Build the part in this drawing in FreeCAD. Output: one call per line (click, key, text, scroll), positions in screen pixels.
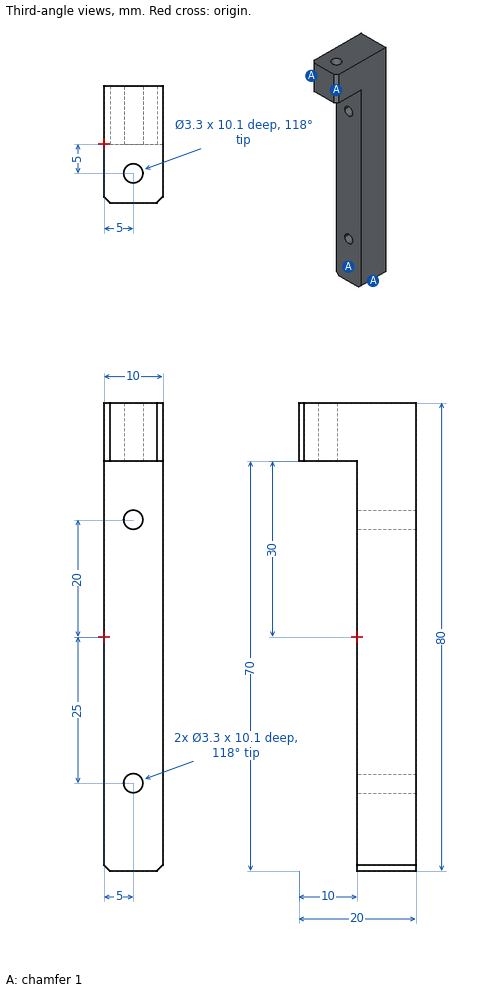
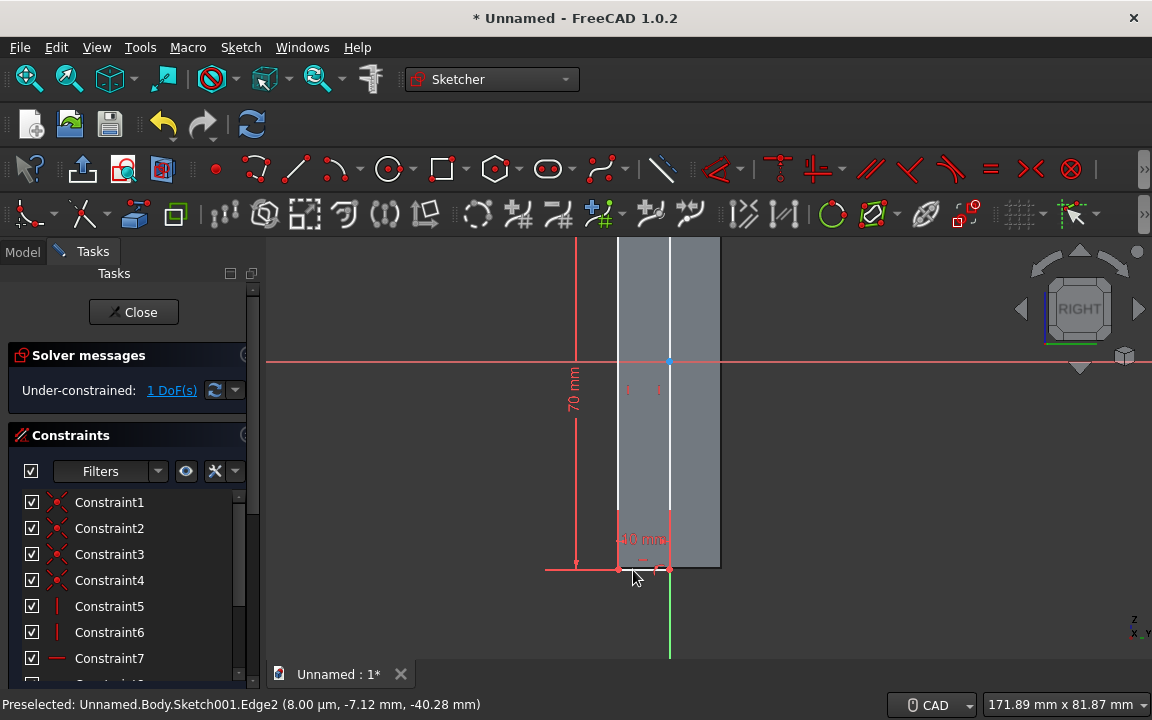
scroll(634, 570, down, 2)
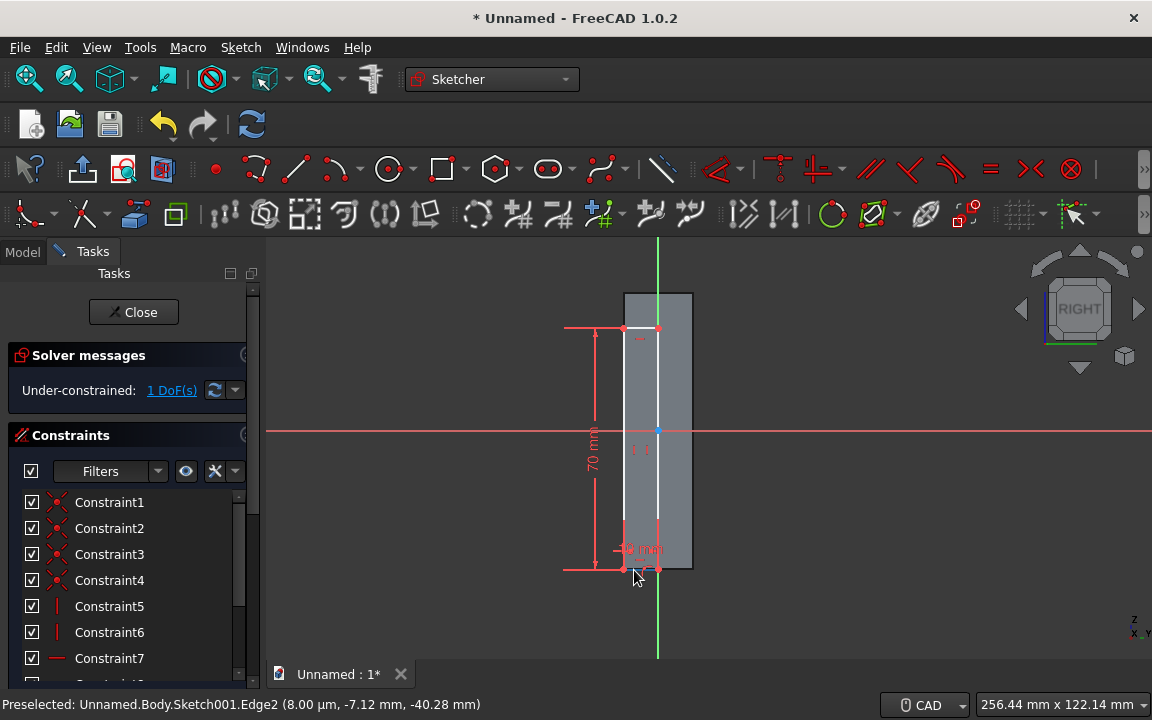
click(624, 328)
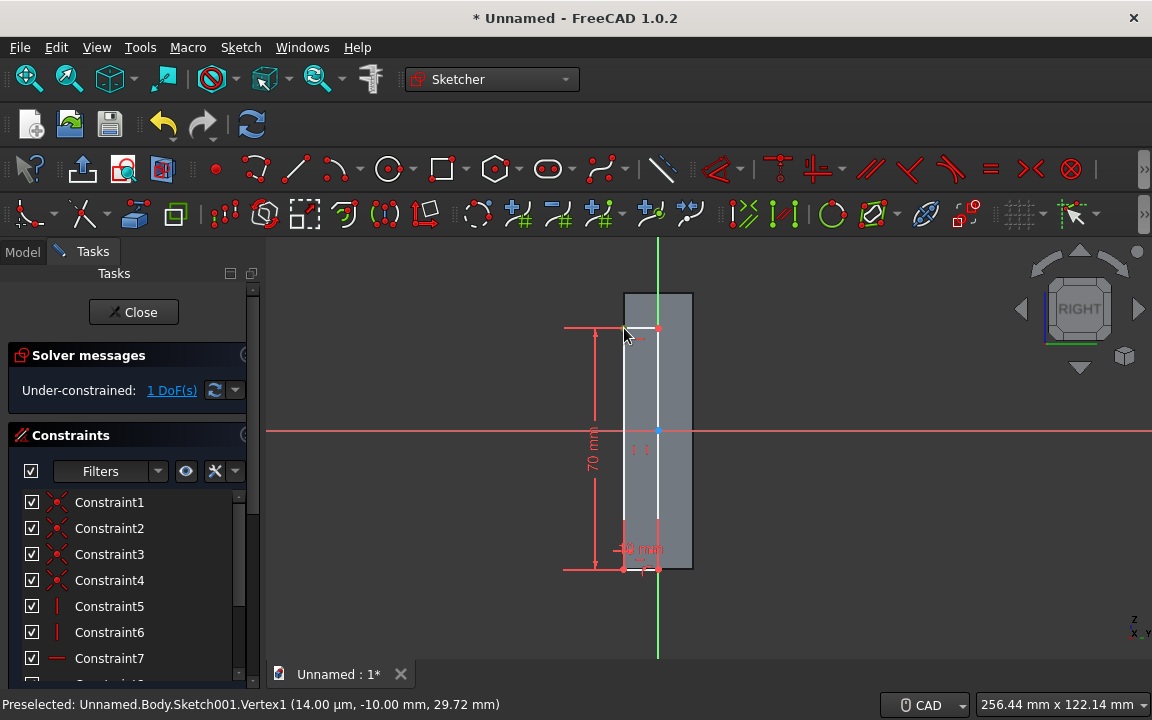
key(i)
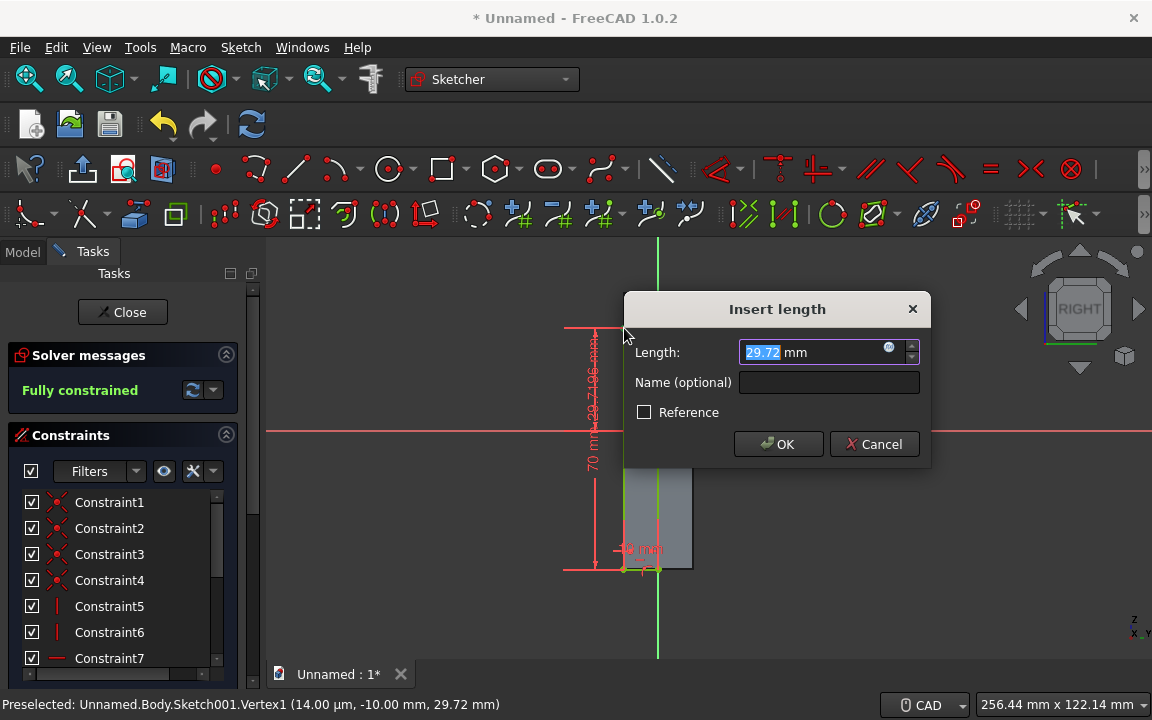
text(30)
key(Return)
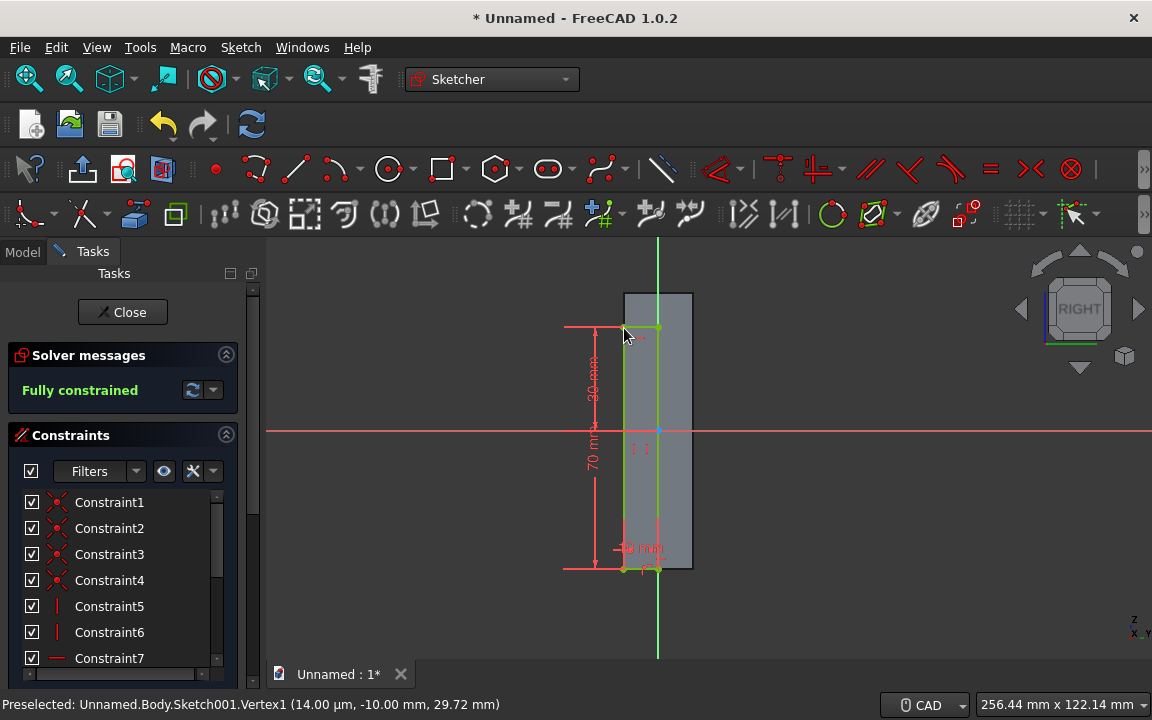
click(123, 312)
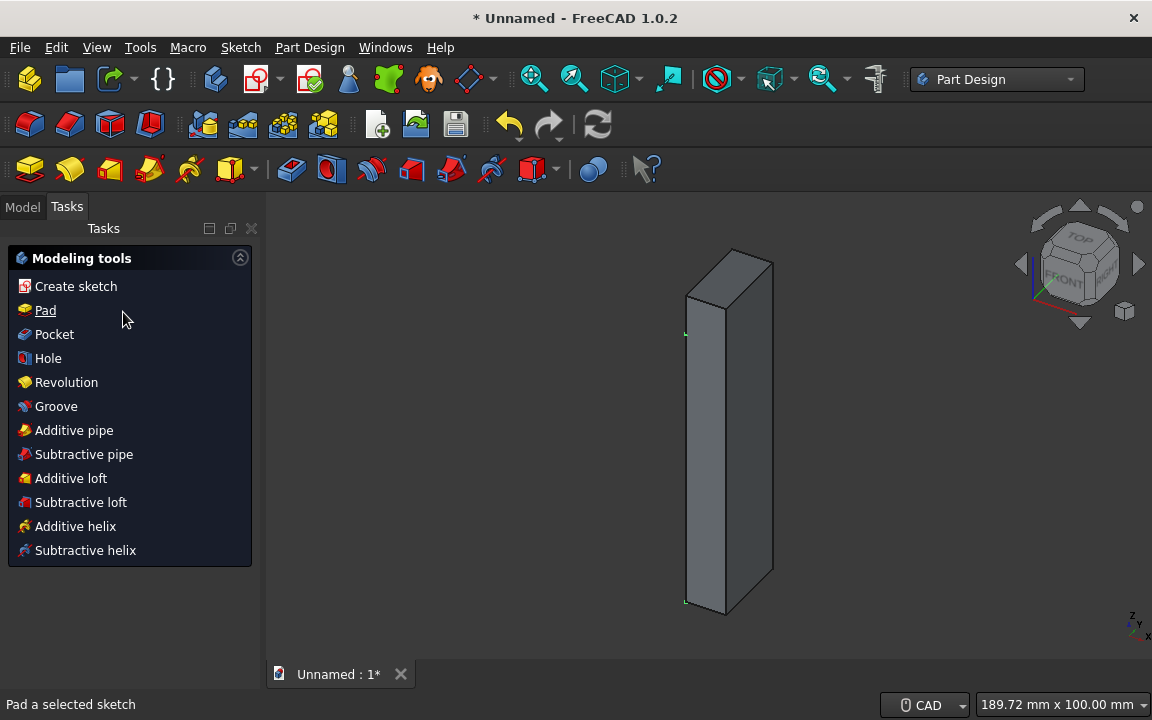
click(292, 170)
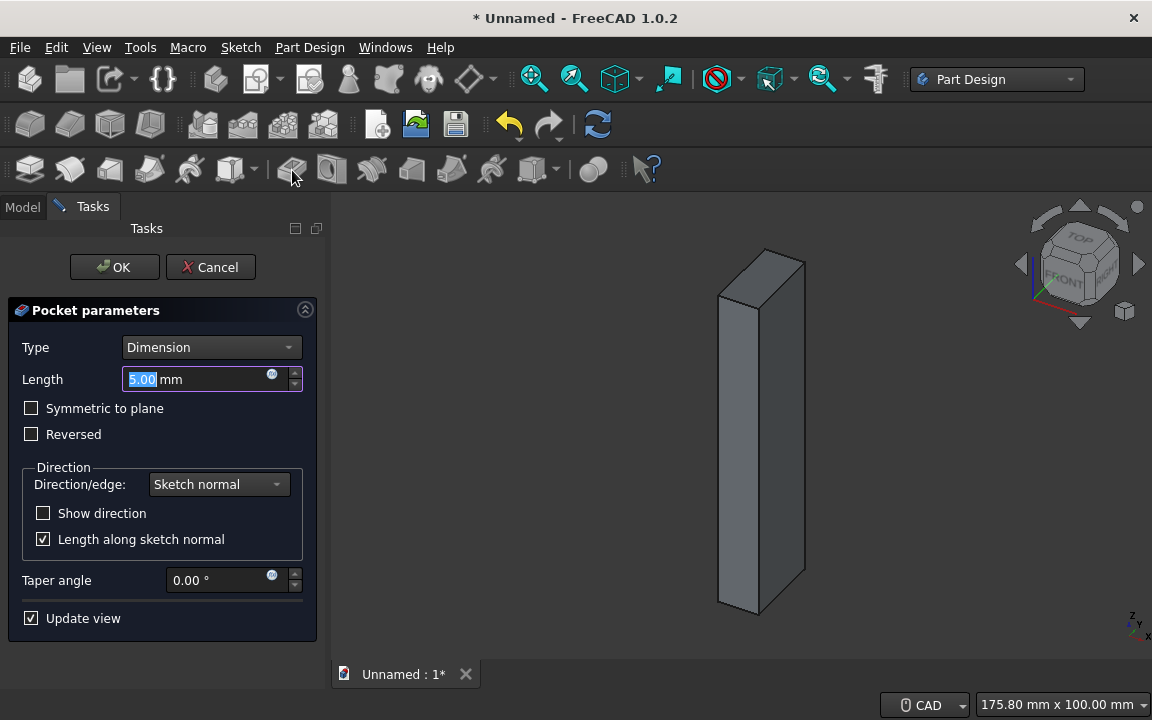
click(212, 348)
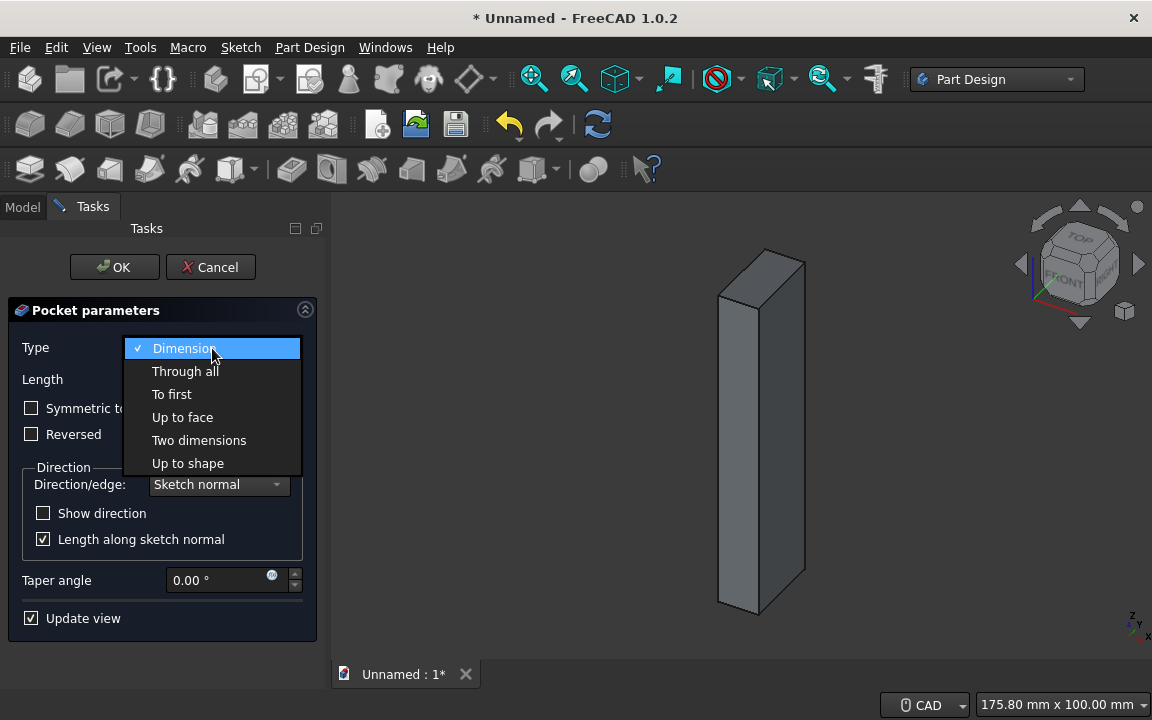
click(212, 372)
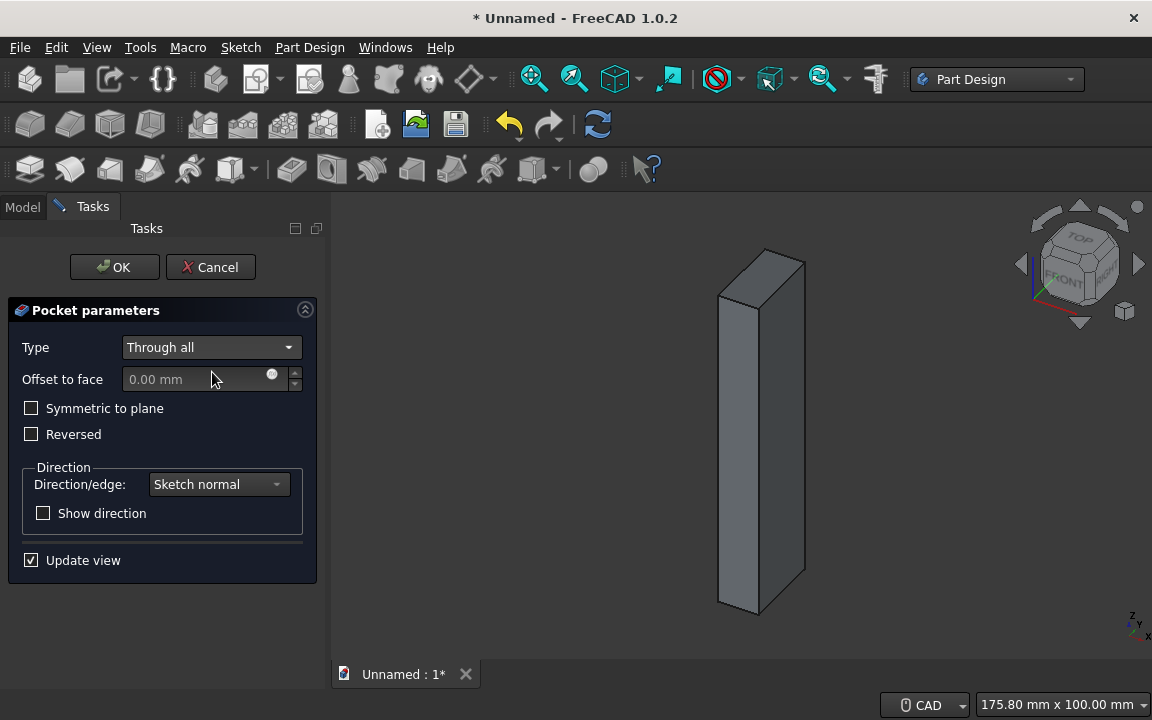
click(30, 434)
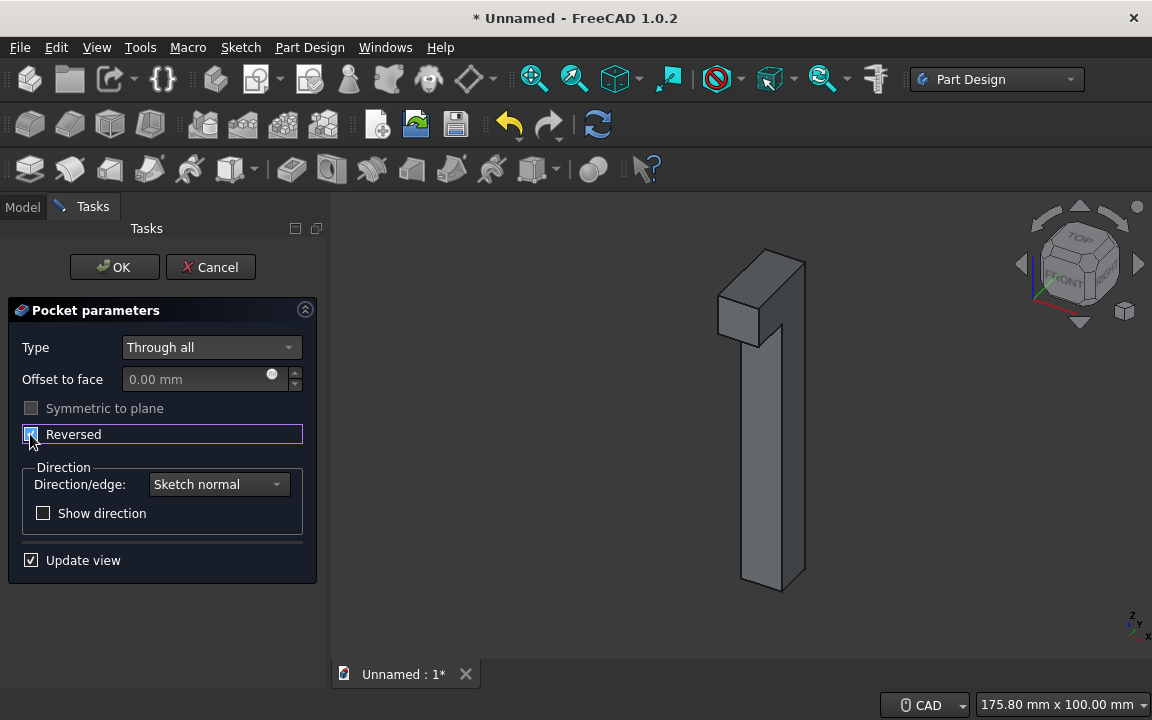
click(115, 267)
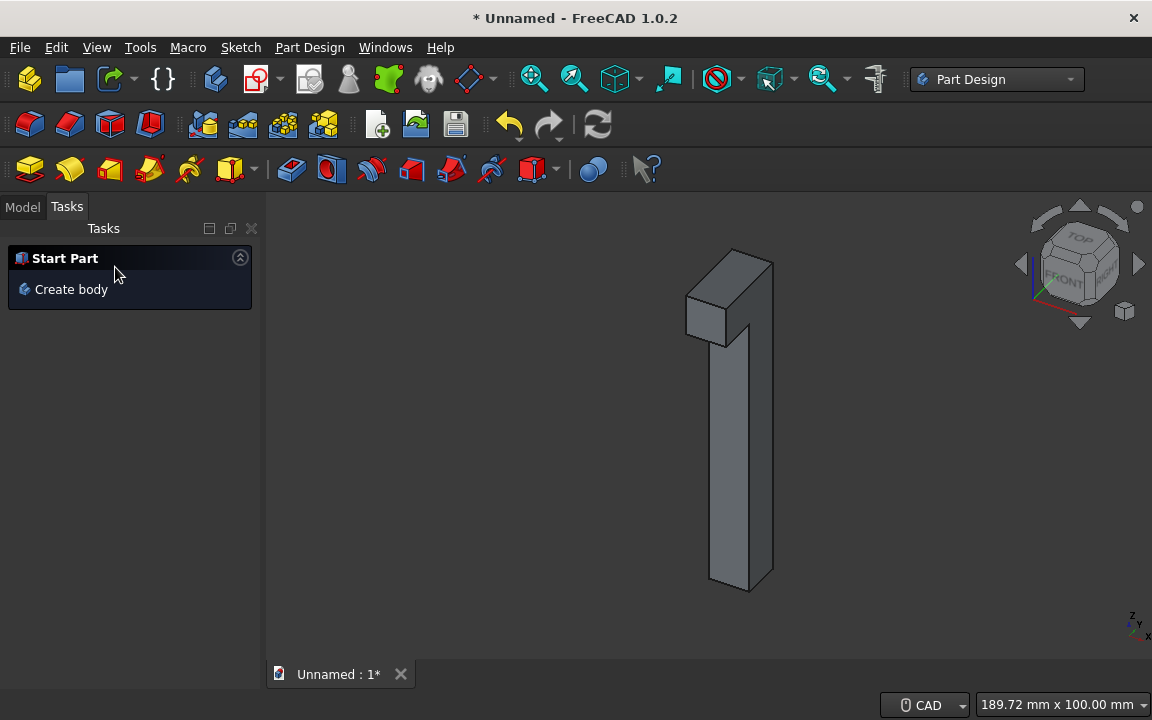
key(5)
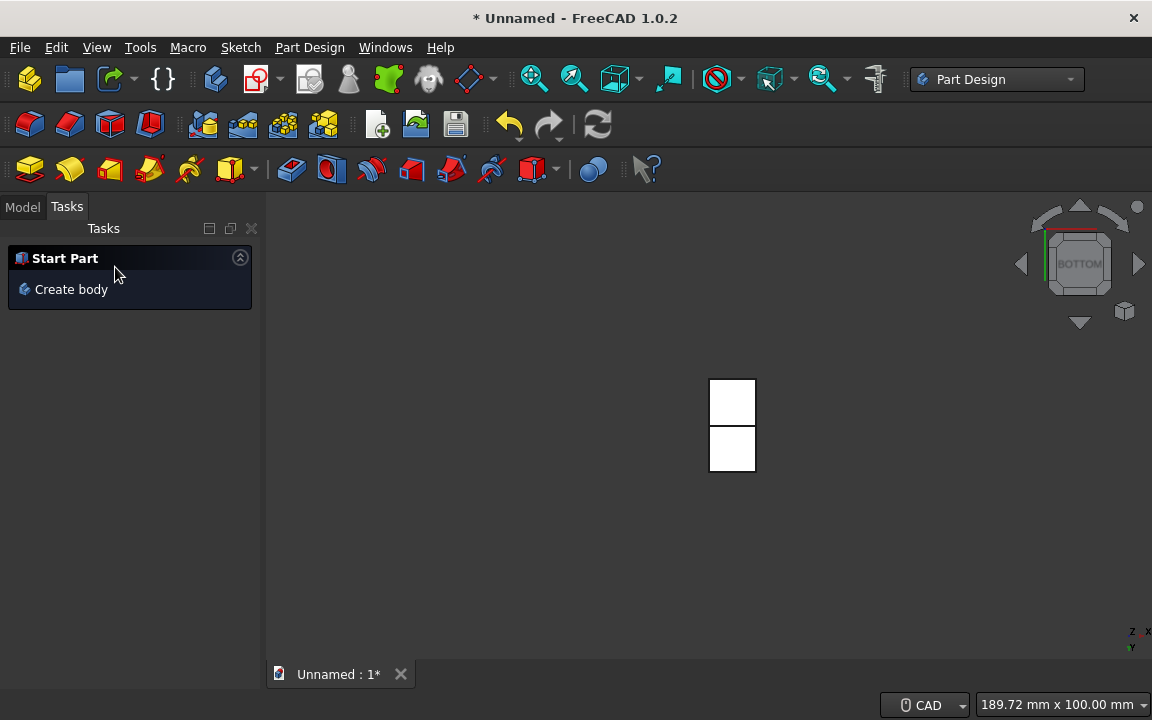
key(v)
key(f)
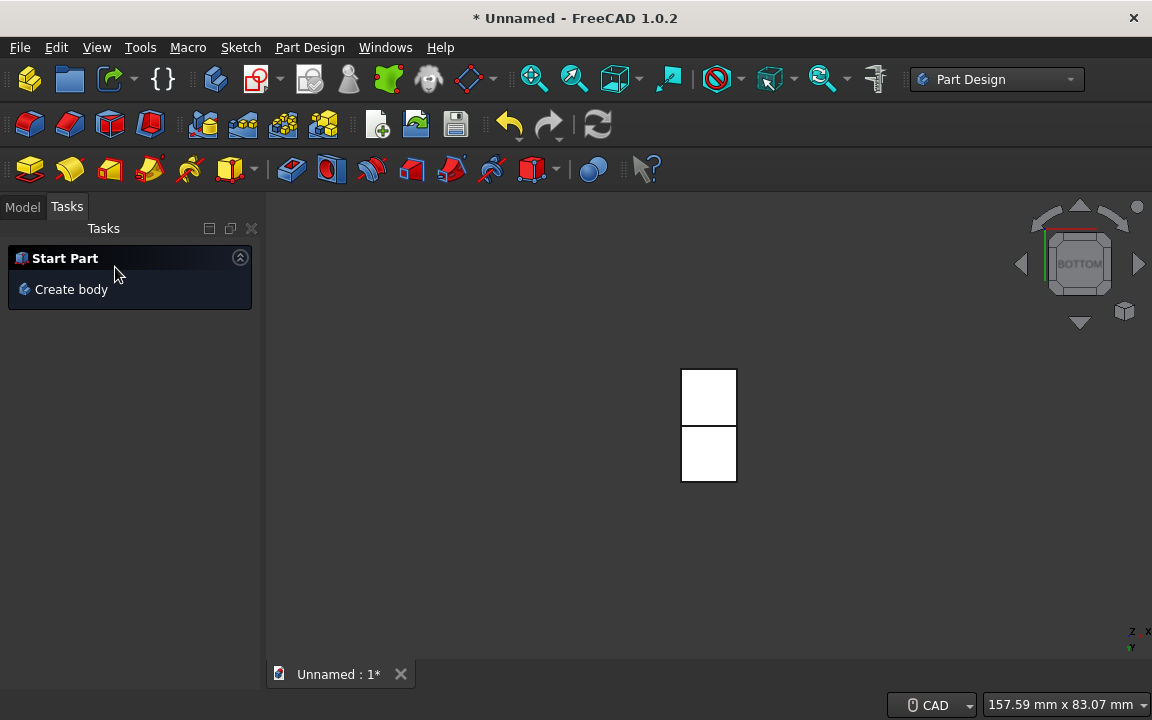
click(709, 396)